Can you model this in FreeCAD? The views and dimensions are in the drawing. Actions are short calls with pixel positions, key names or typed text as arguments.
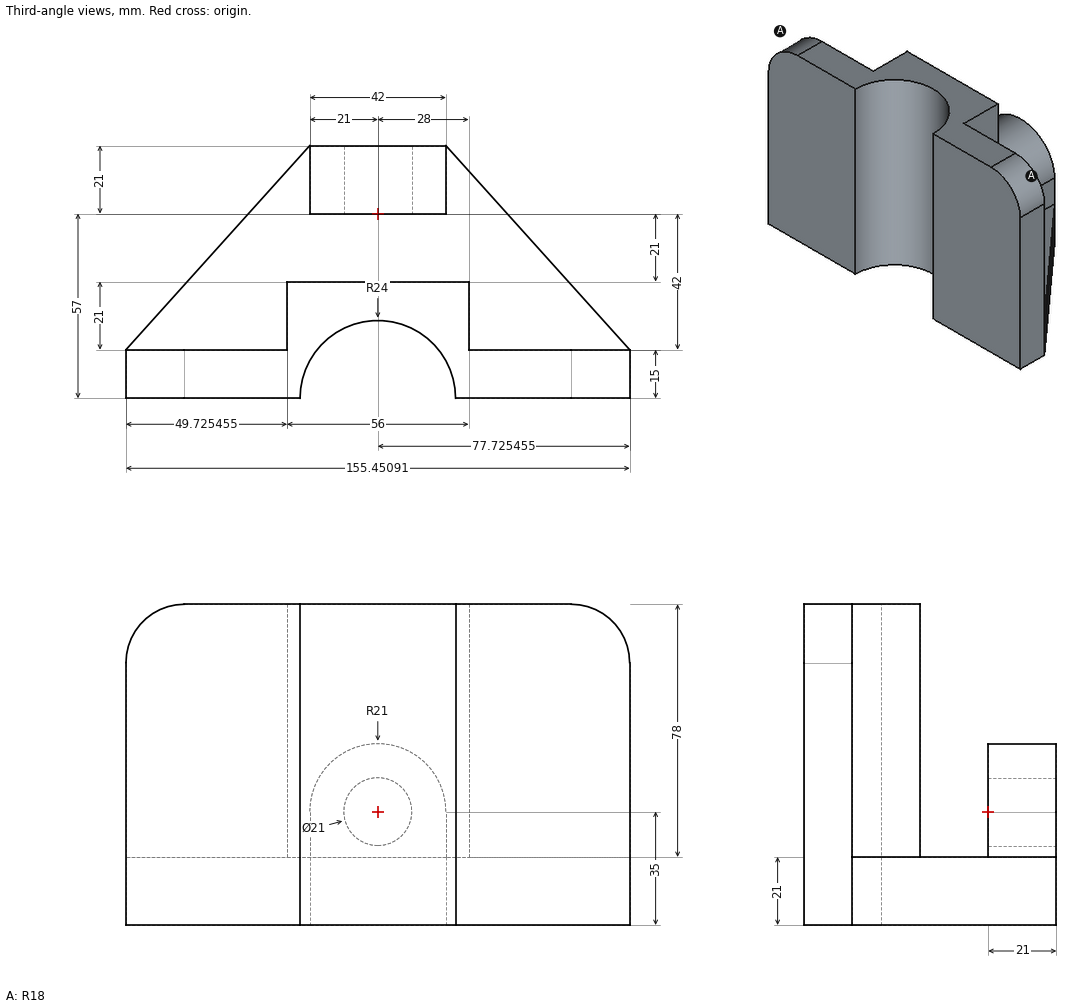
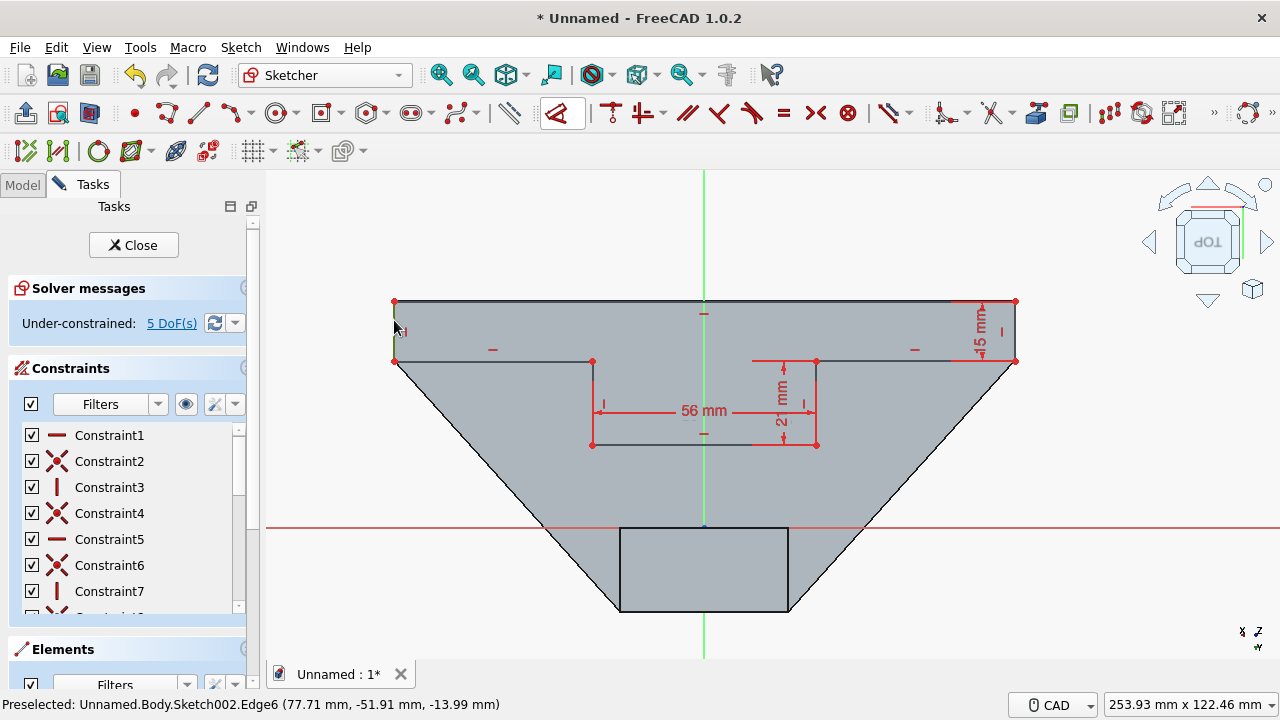
key(i)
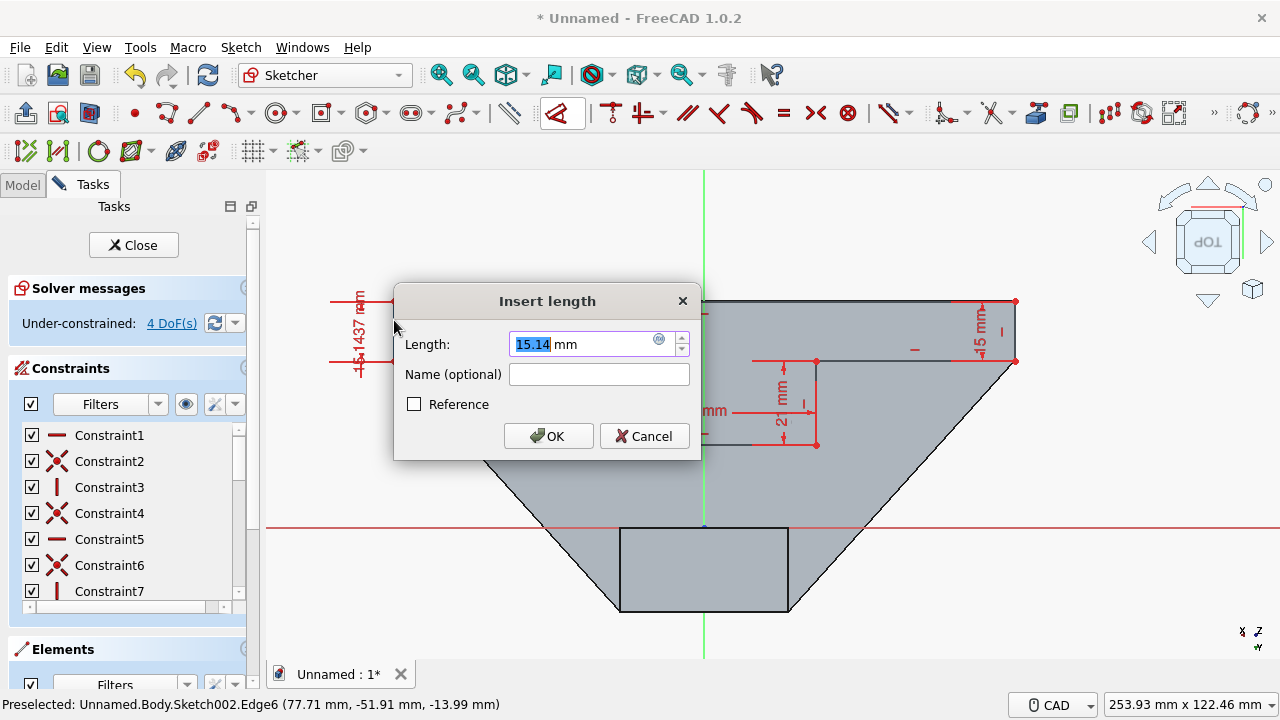
text(15)
key(Return)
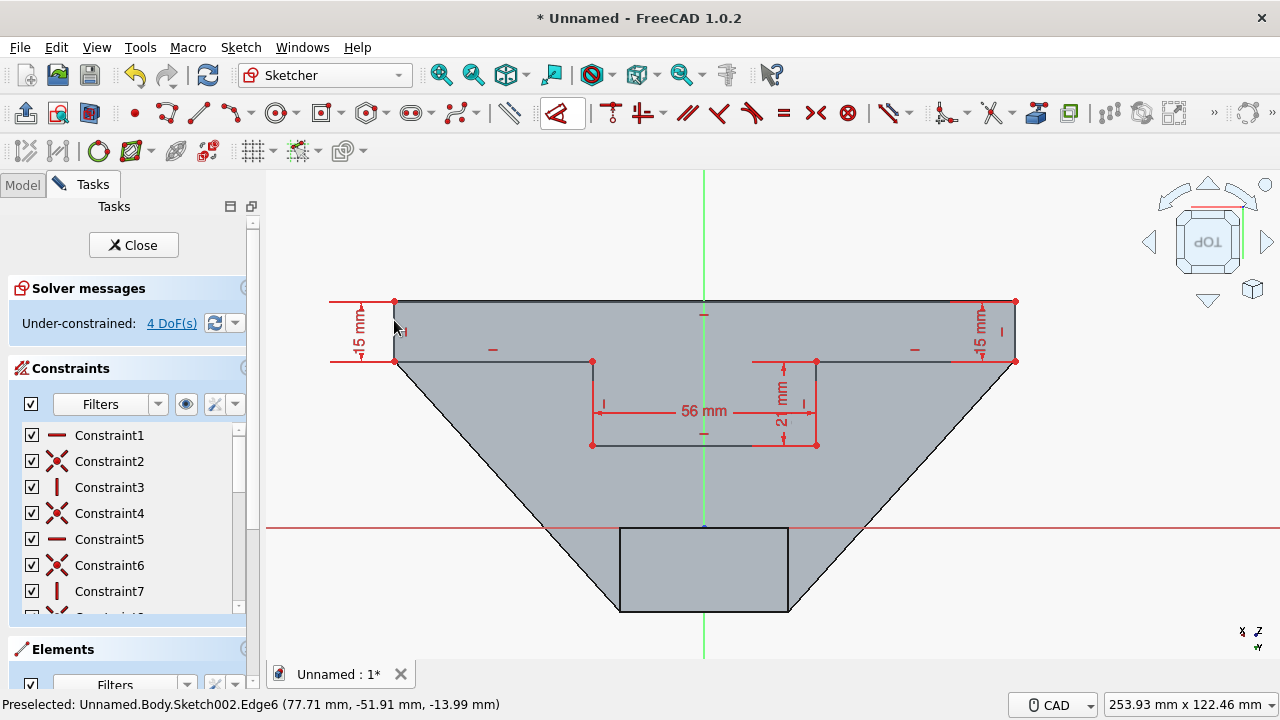
click(593, 446)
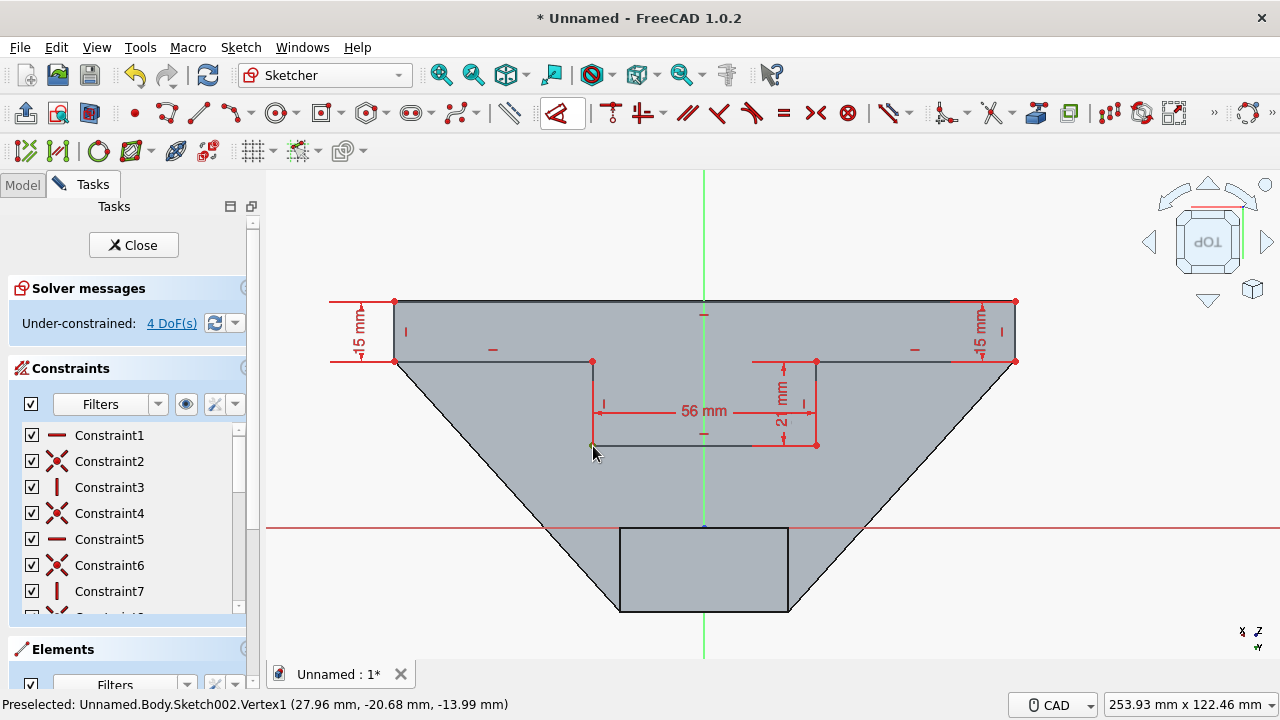
key(l)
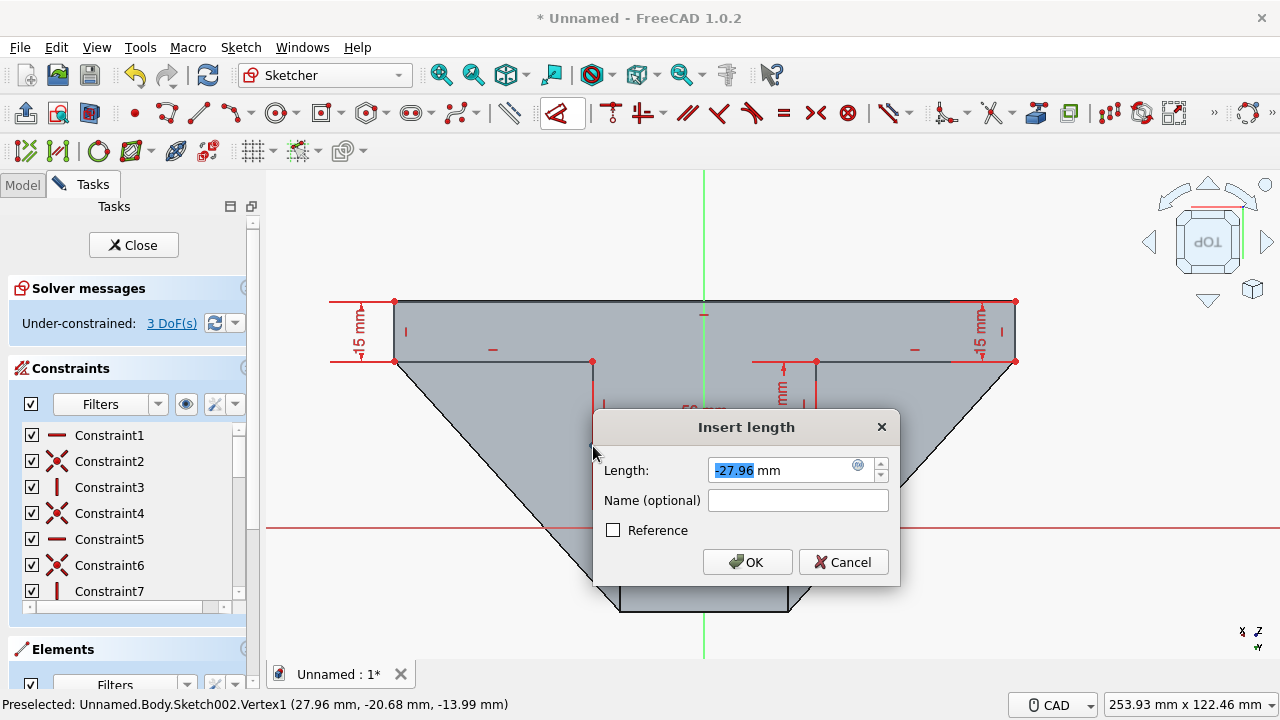
text(-28)
key(Return)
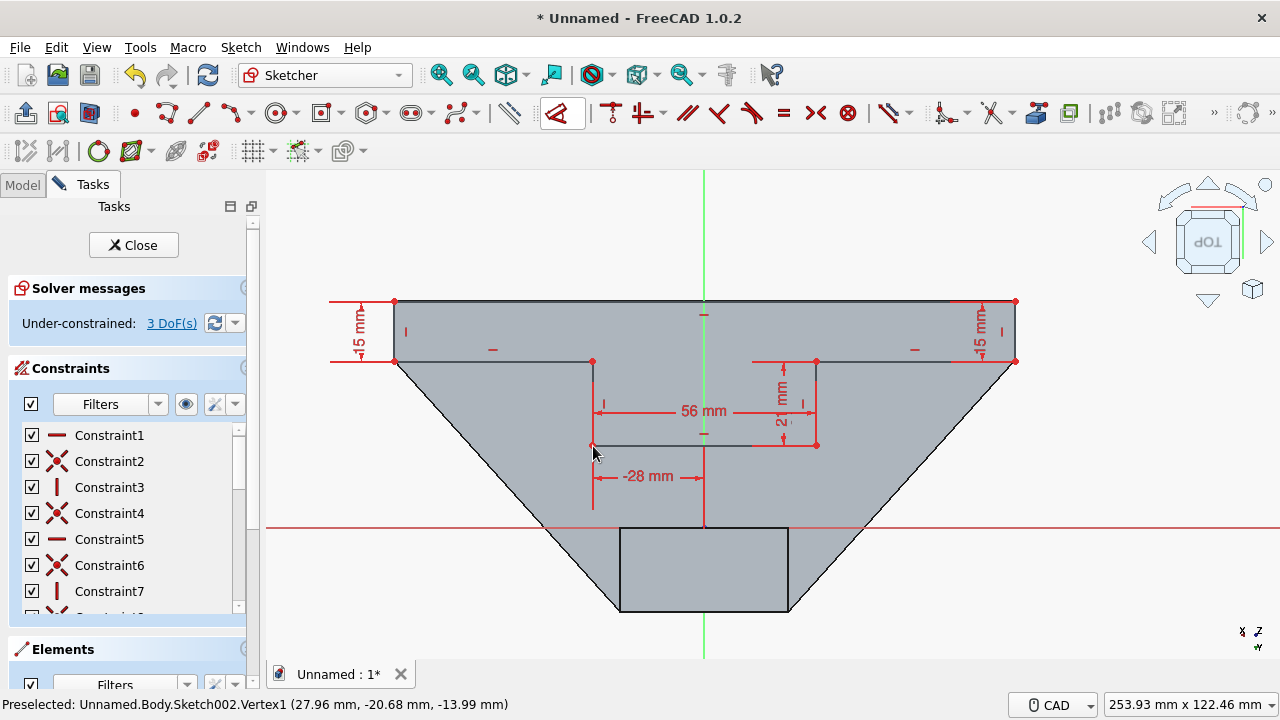
click(593, 446)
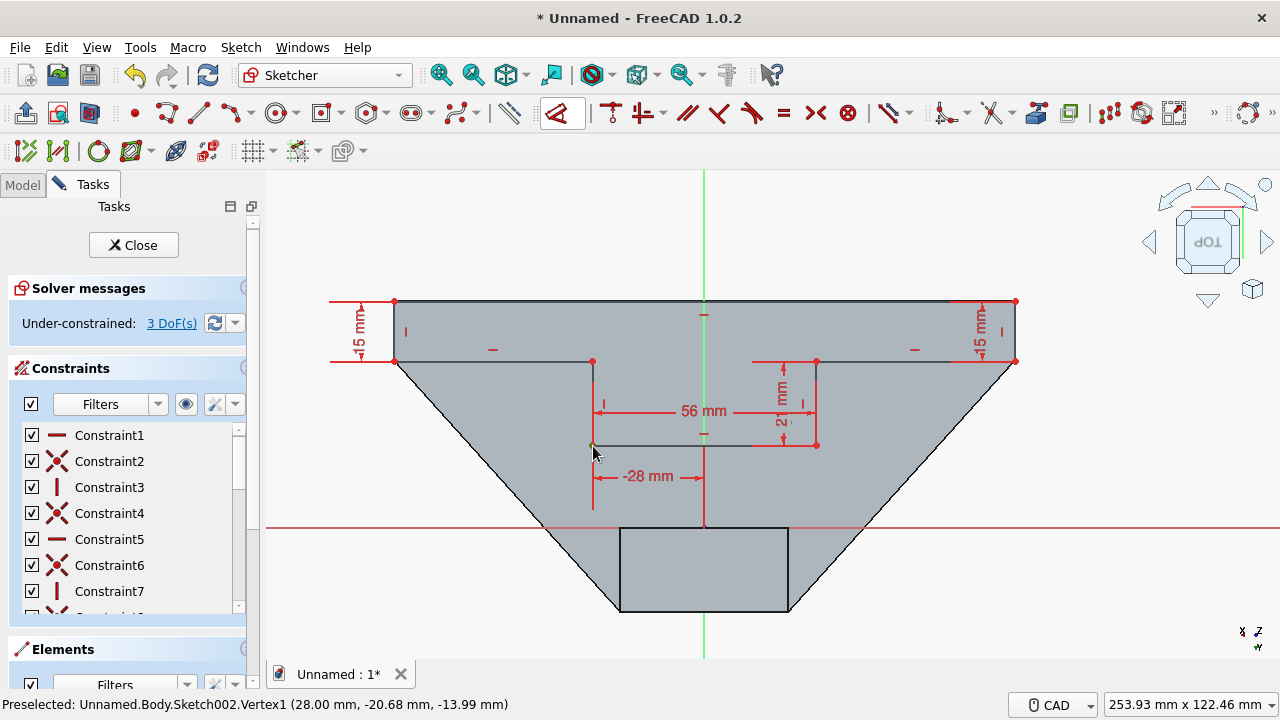
click(580, 114)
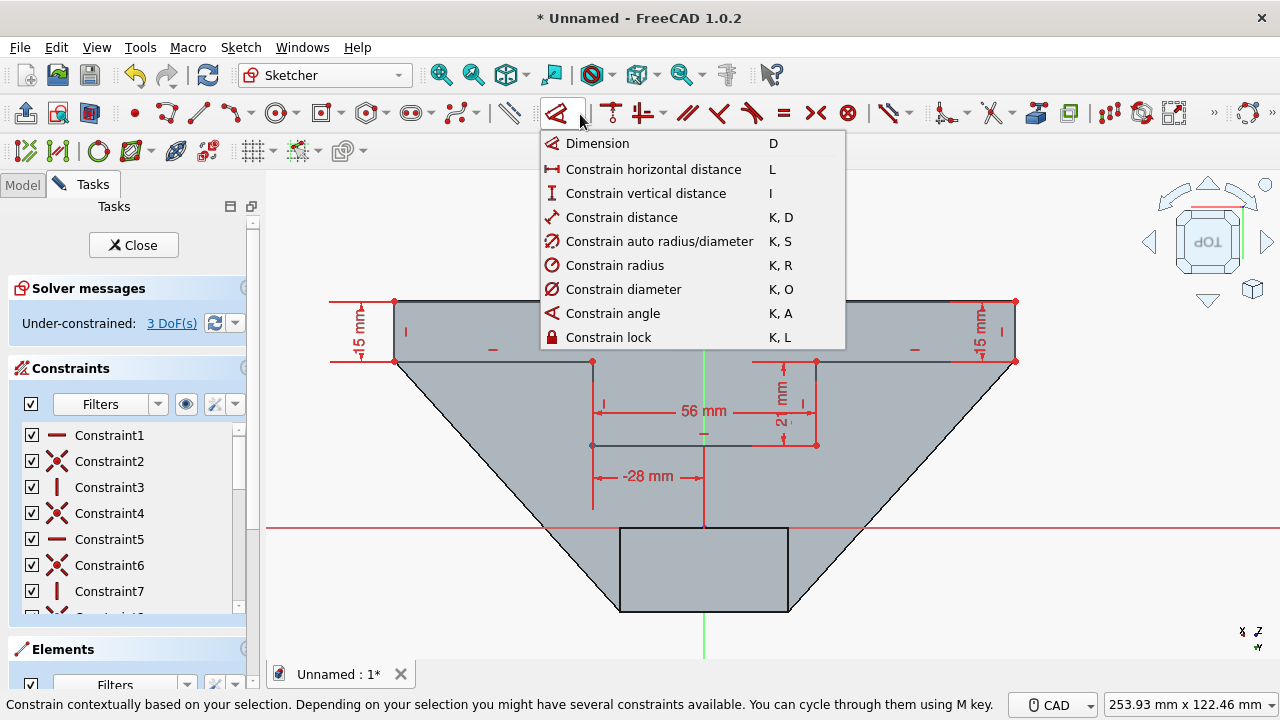
click(693, 193)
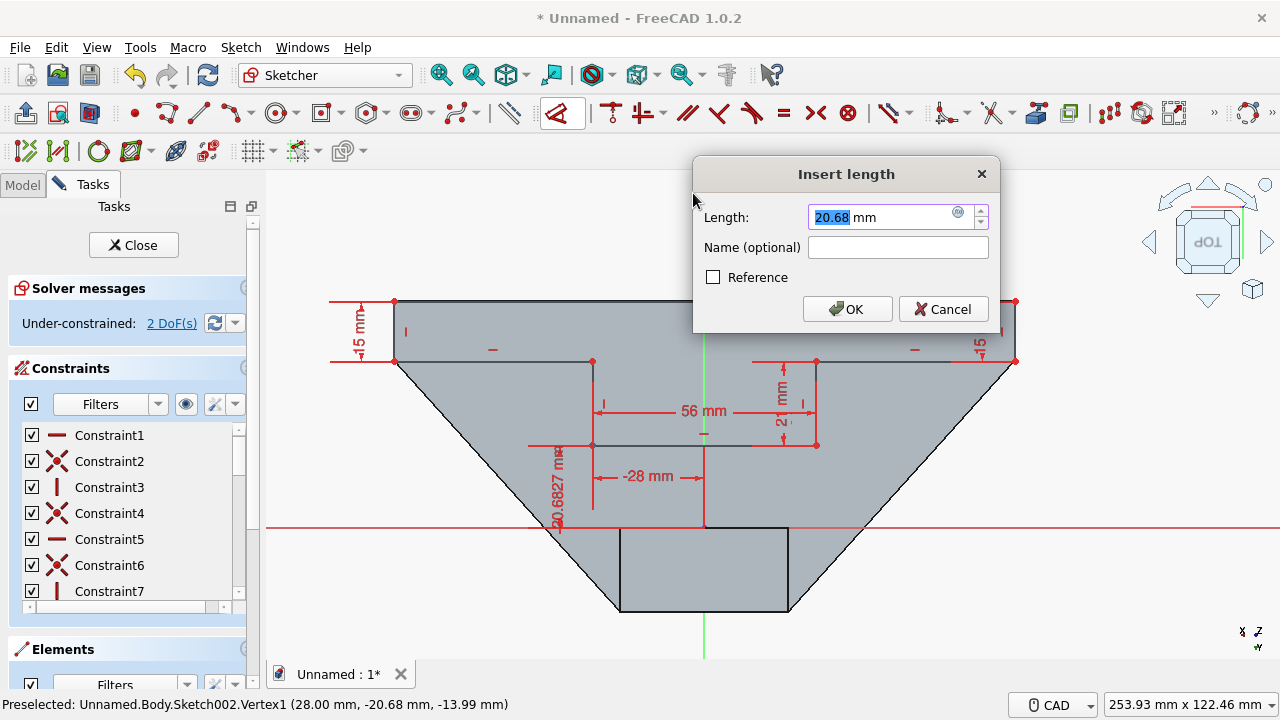
text(21)
key(Return)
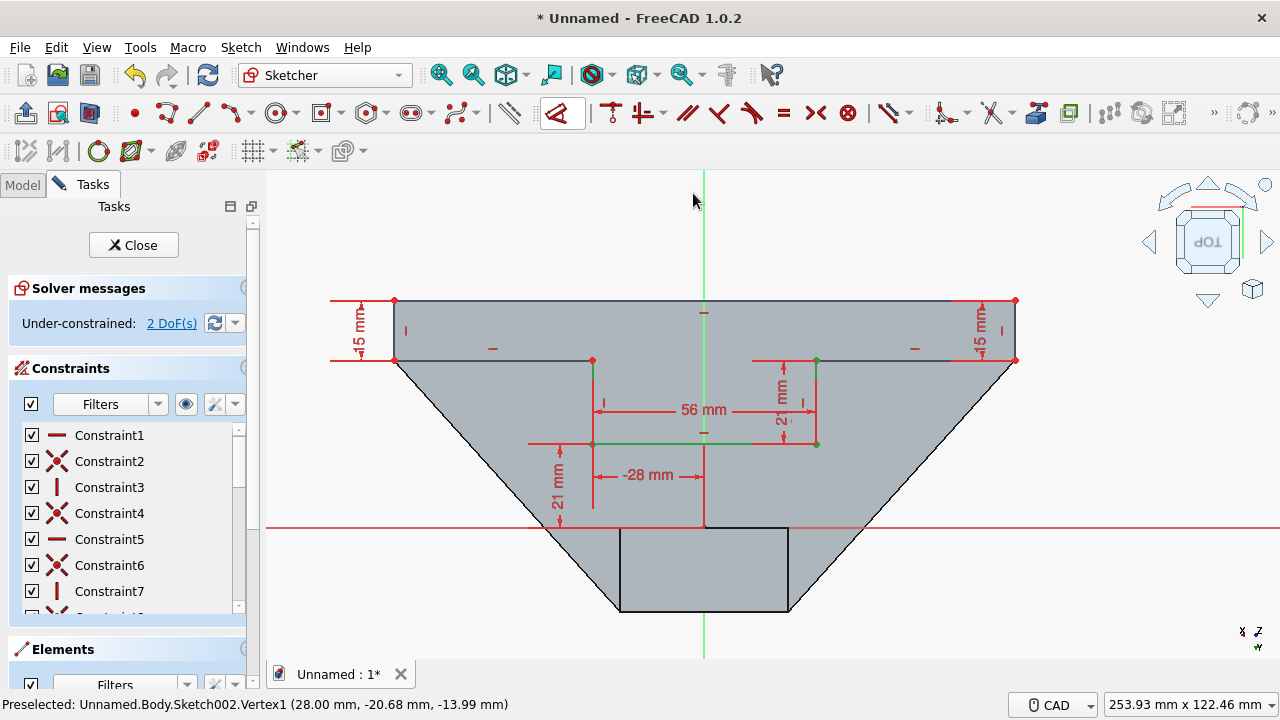
click(876, 361)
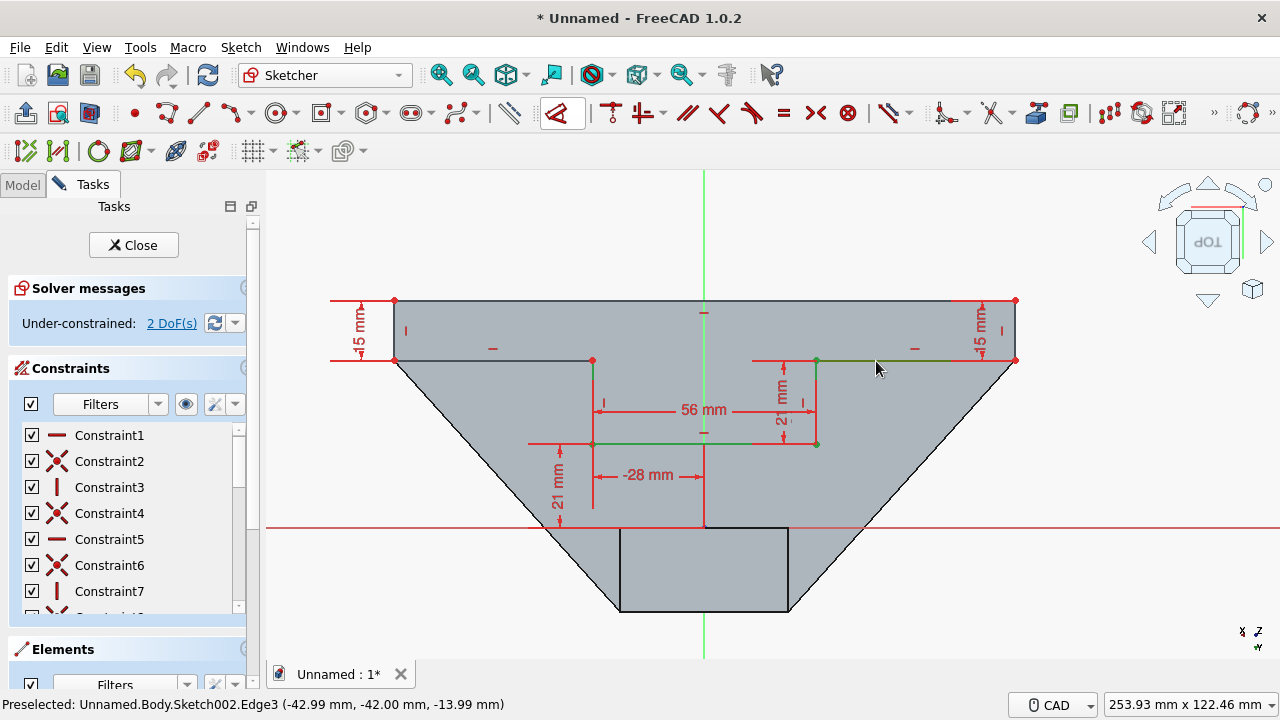
key(l)